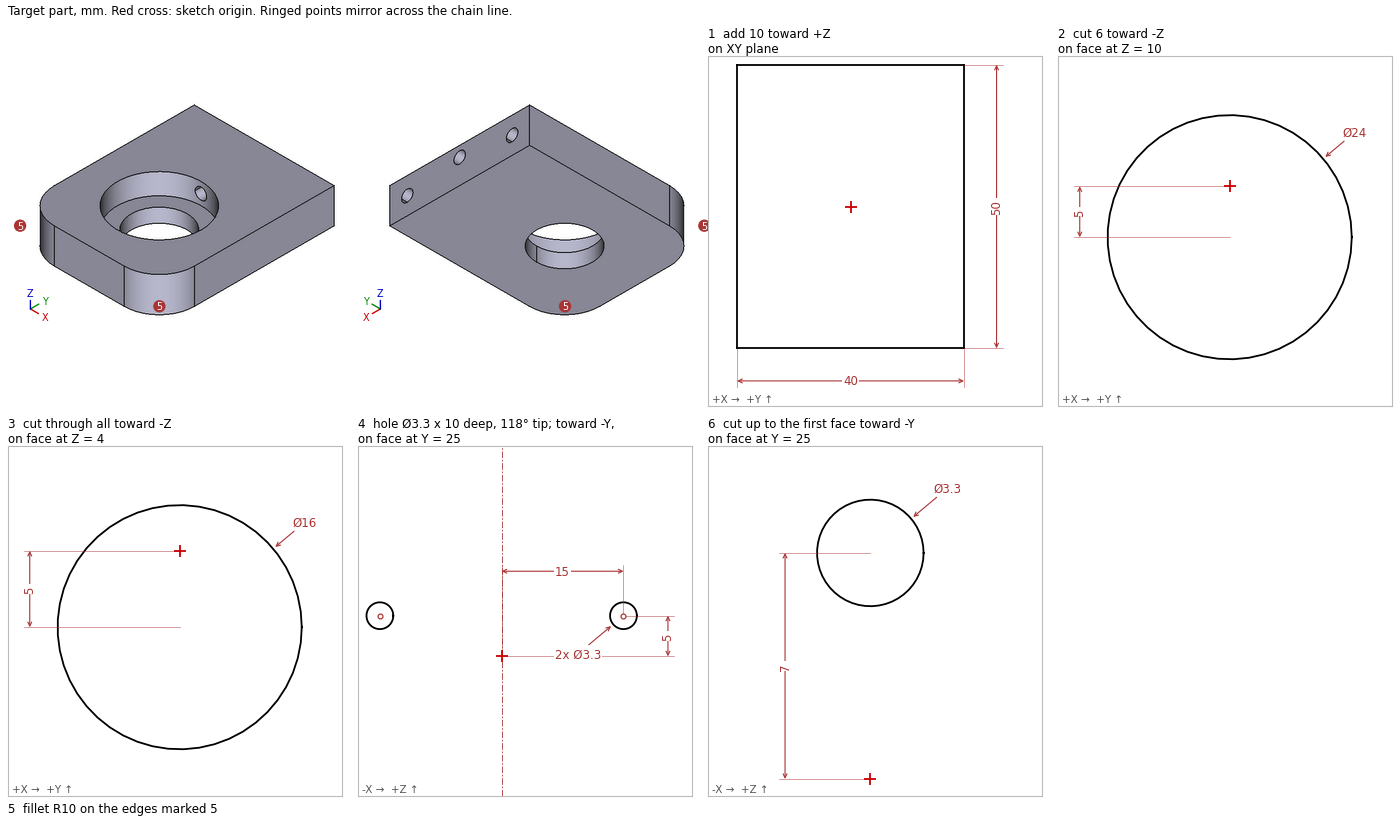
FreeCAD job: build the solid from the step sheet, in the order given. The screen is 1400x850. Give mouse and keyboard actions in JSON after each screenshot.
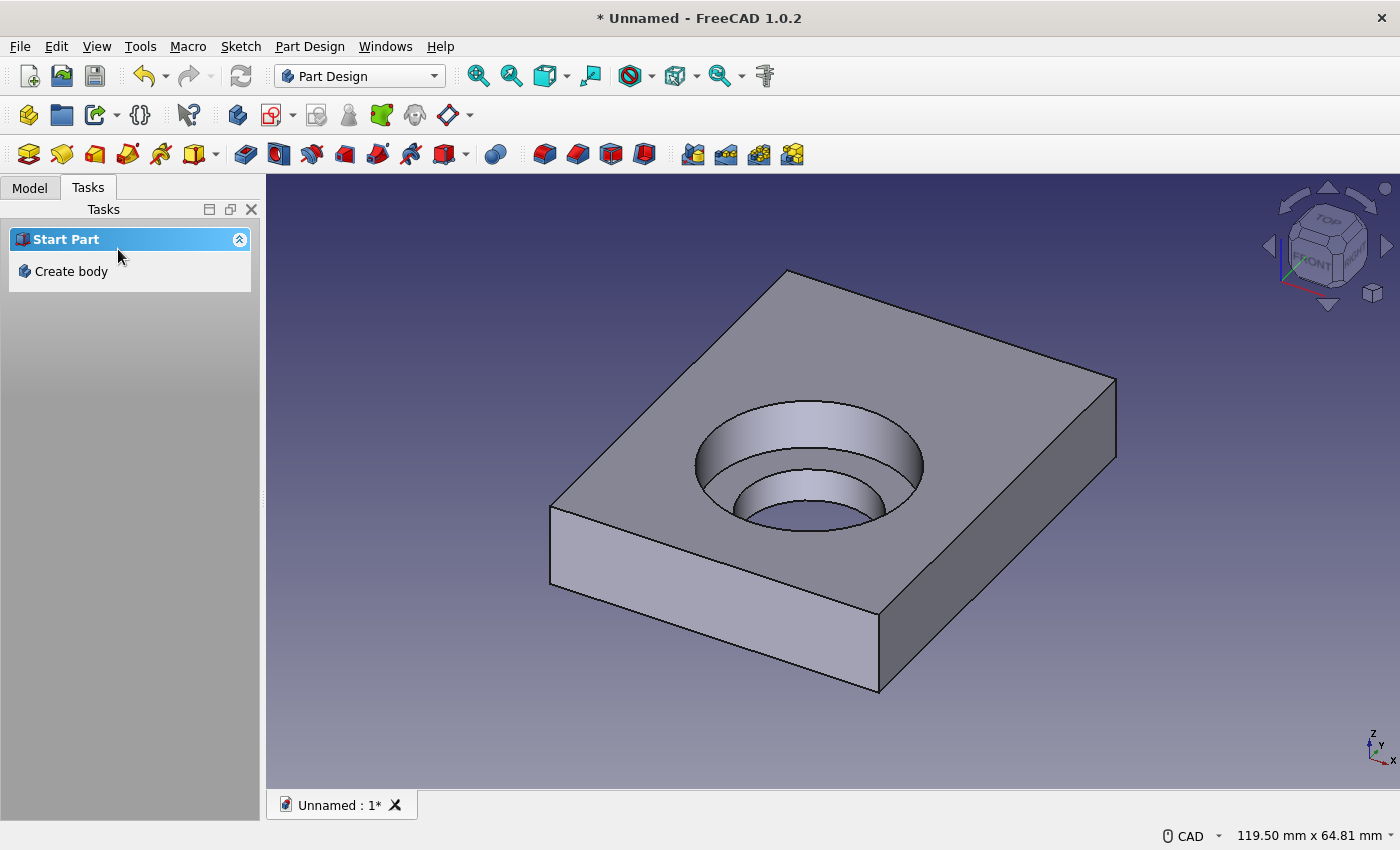
{"action": "key", "text": "4"}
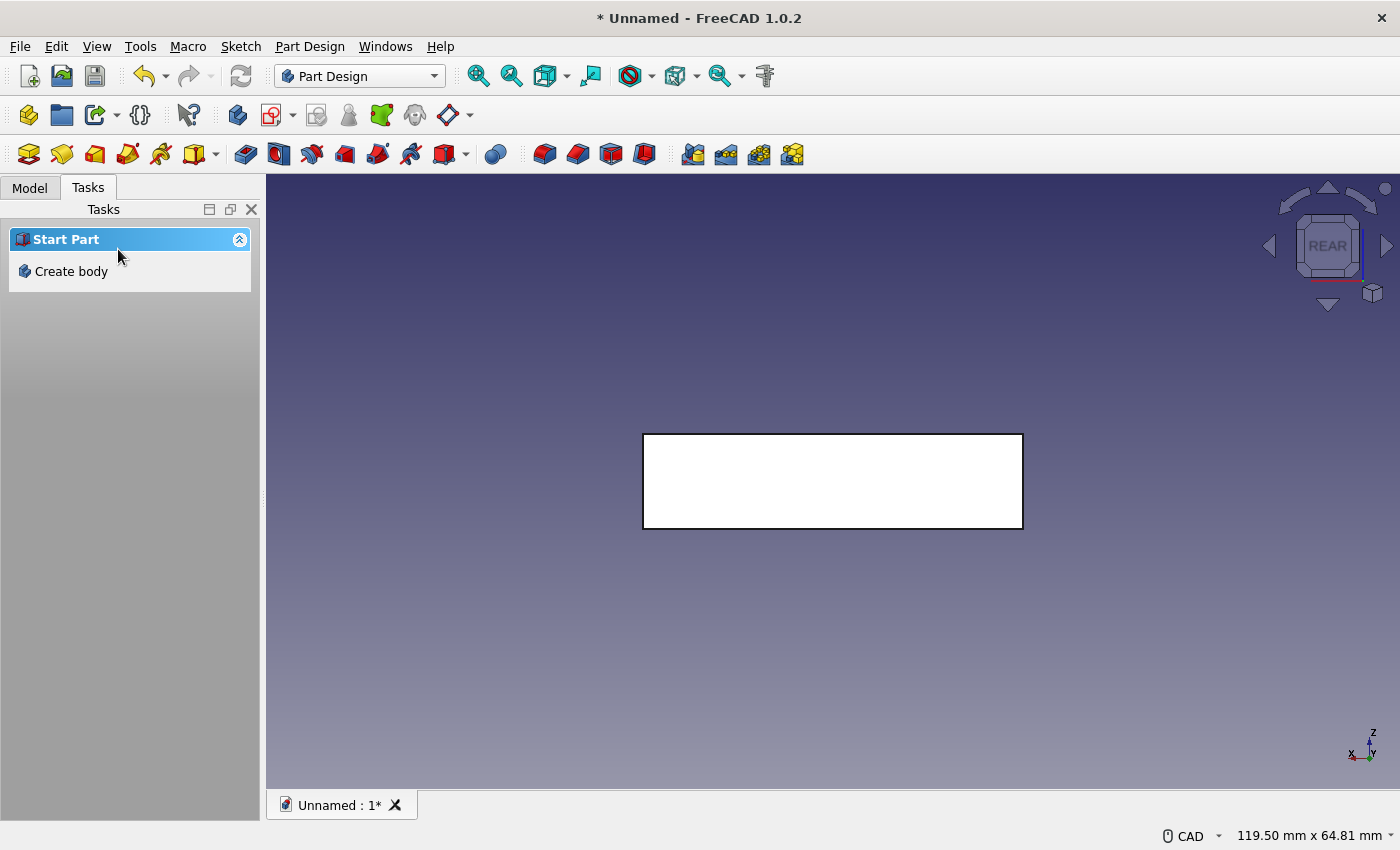
{"action": "left_click", "coordinate": [479, 76]}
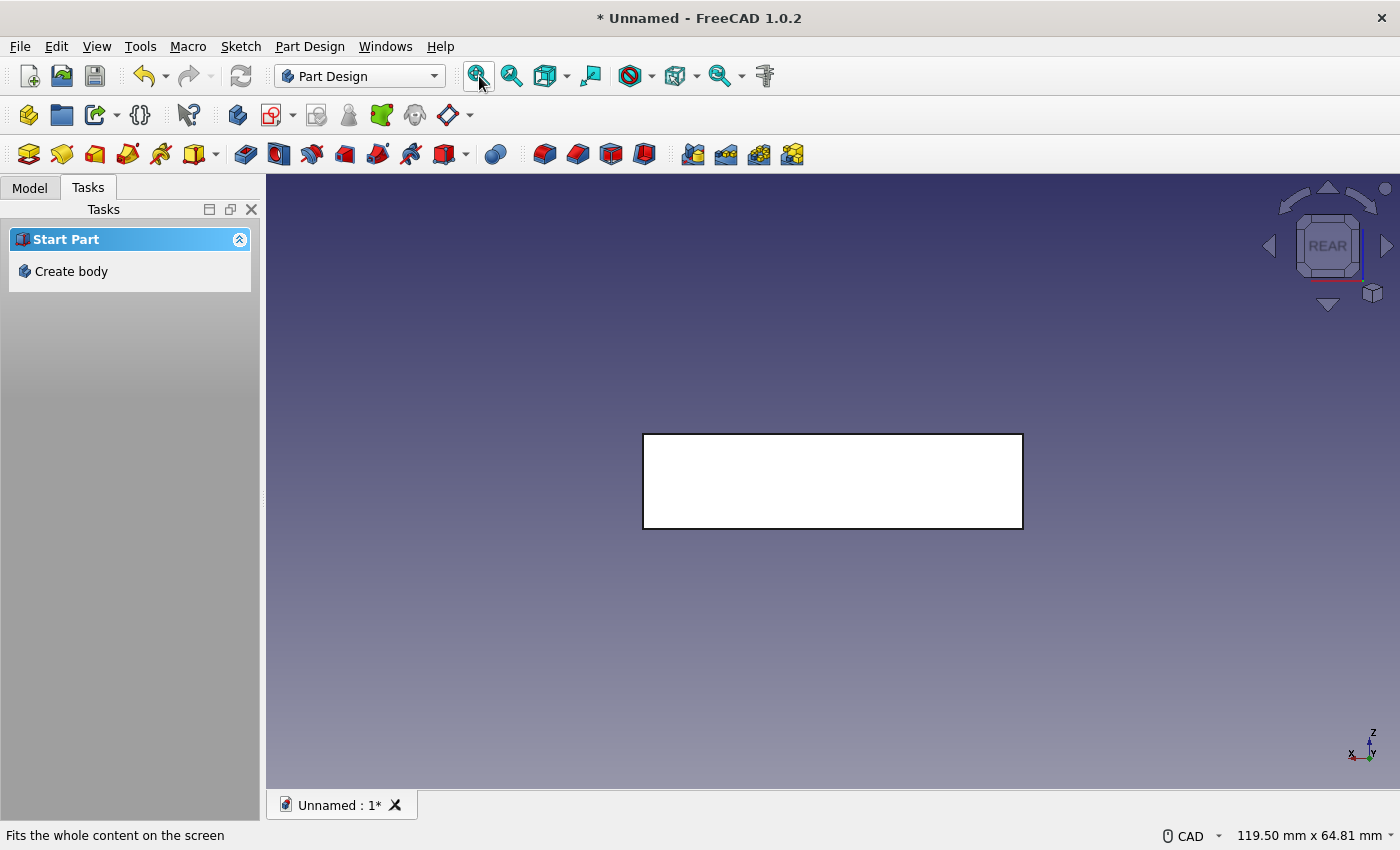
{"action": "left_click", "coordinate": [725, 481]}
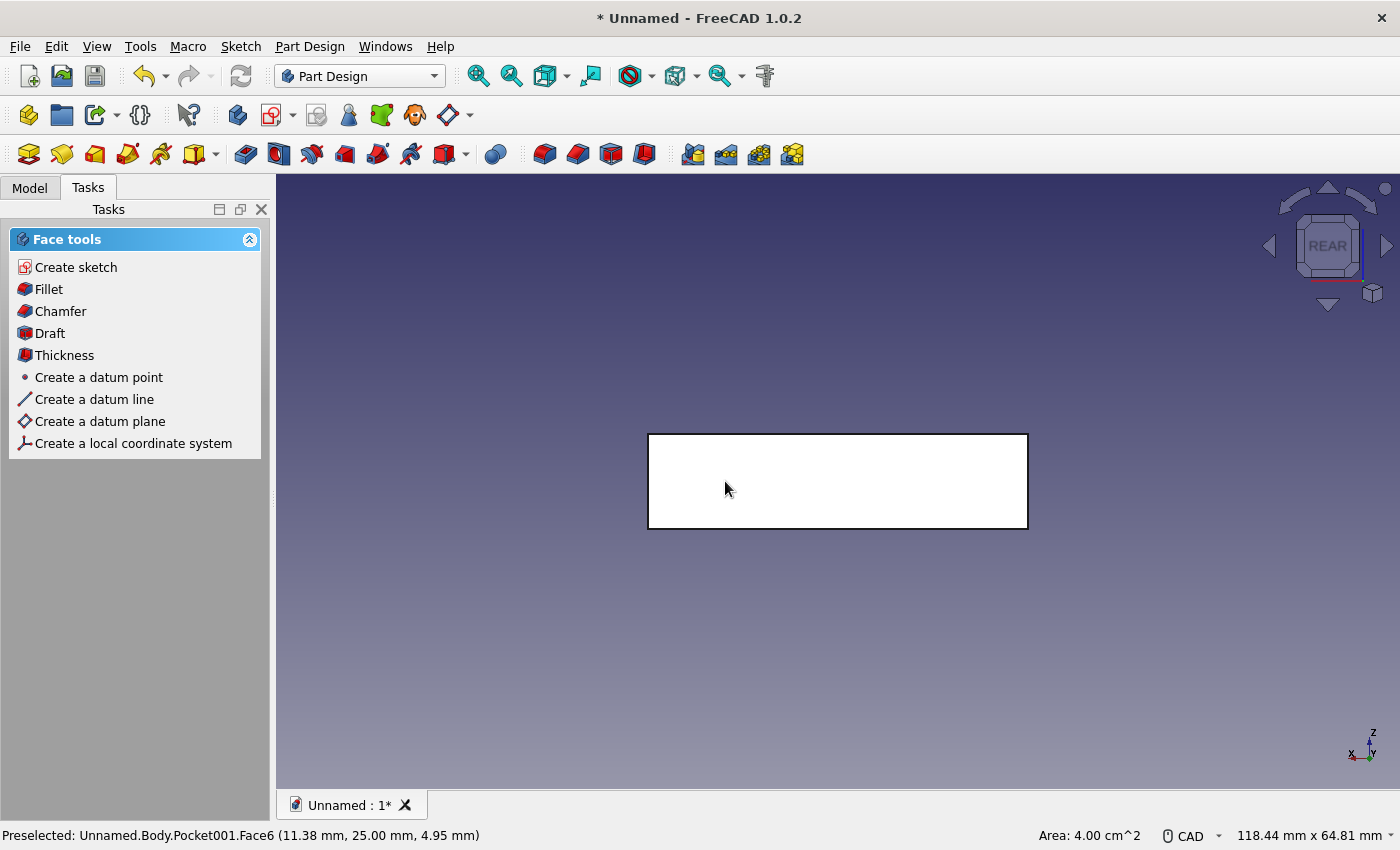
{"action": "left_click", "coordinate": [270, 116]}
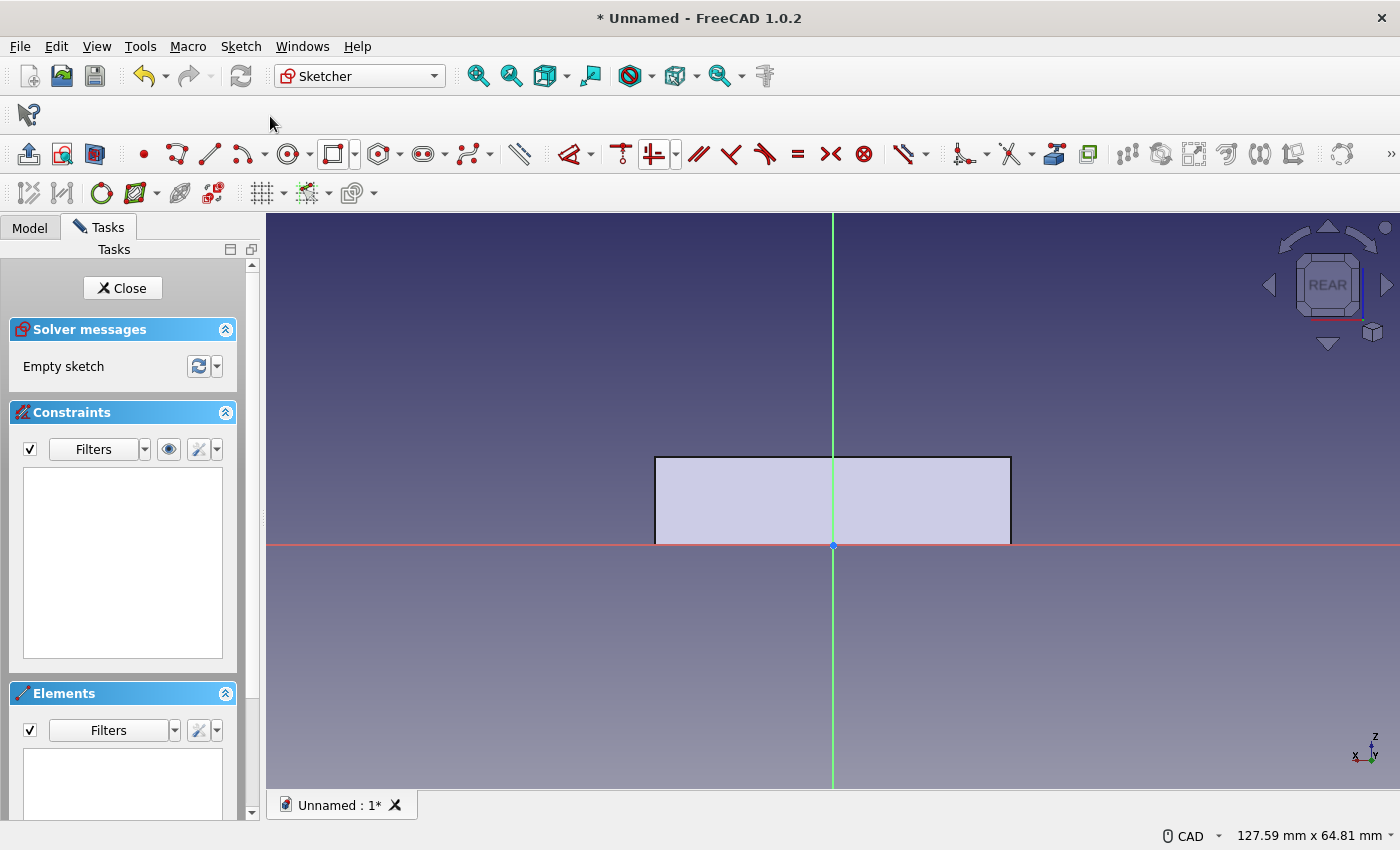
{"action": "scroll", "coordinate": [889, 528], "scroll_direction": "up", "scroll_amount": 4}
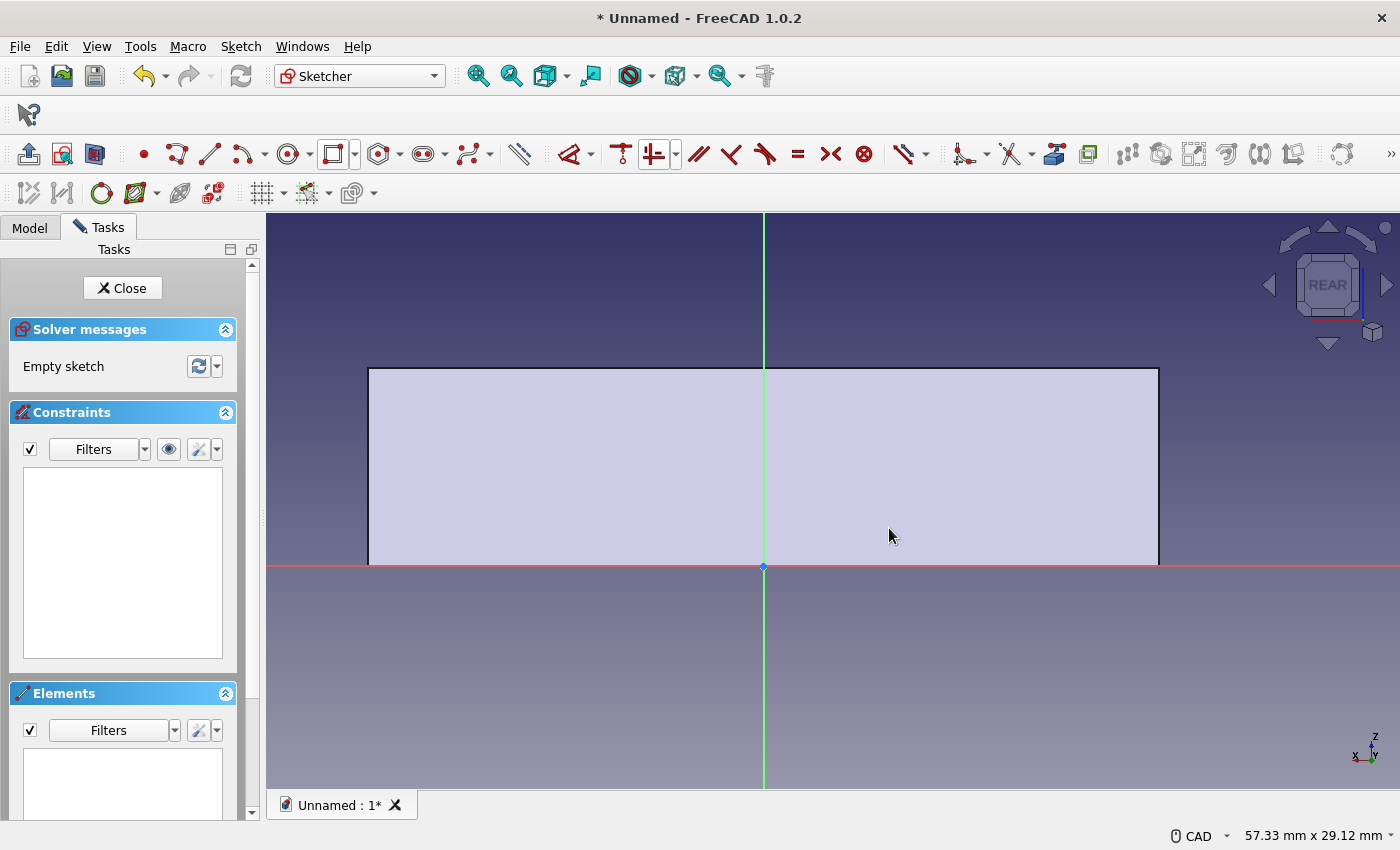
{"action": "left_click", "coordinate": [288, 154]}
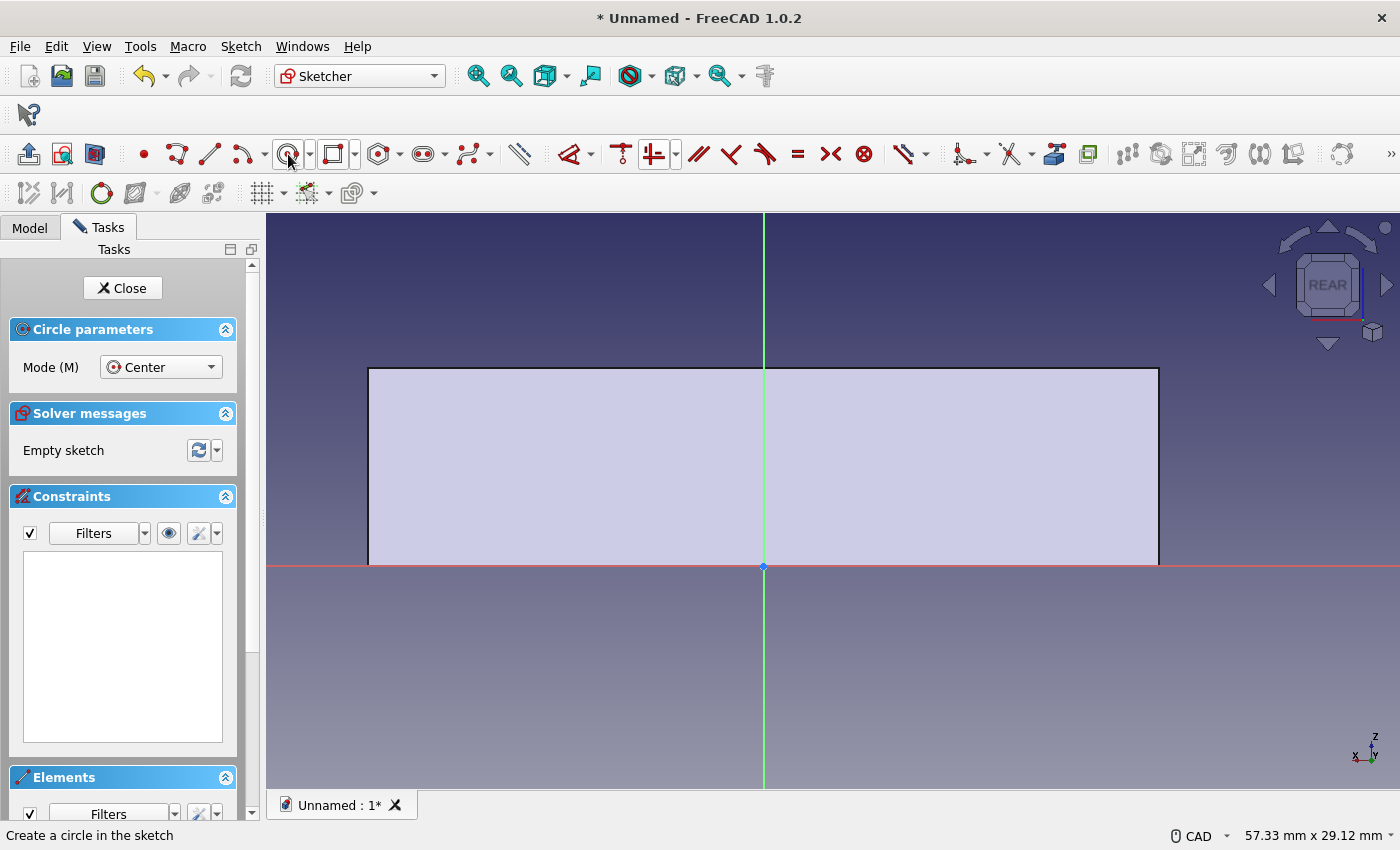
{"action": "left_click", "coordinate": [1060, 467]}
{"action": "mouse_move", "coordinate": [1083, 444]}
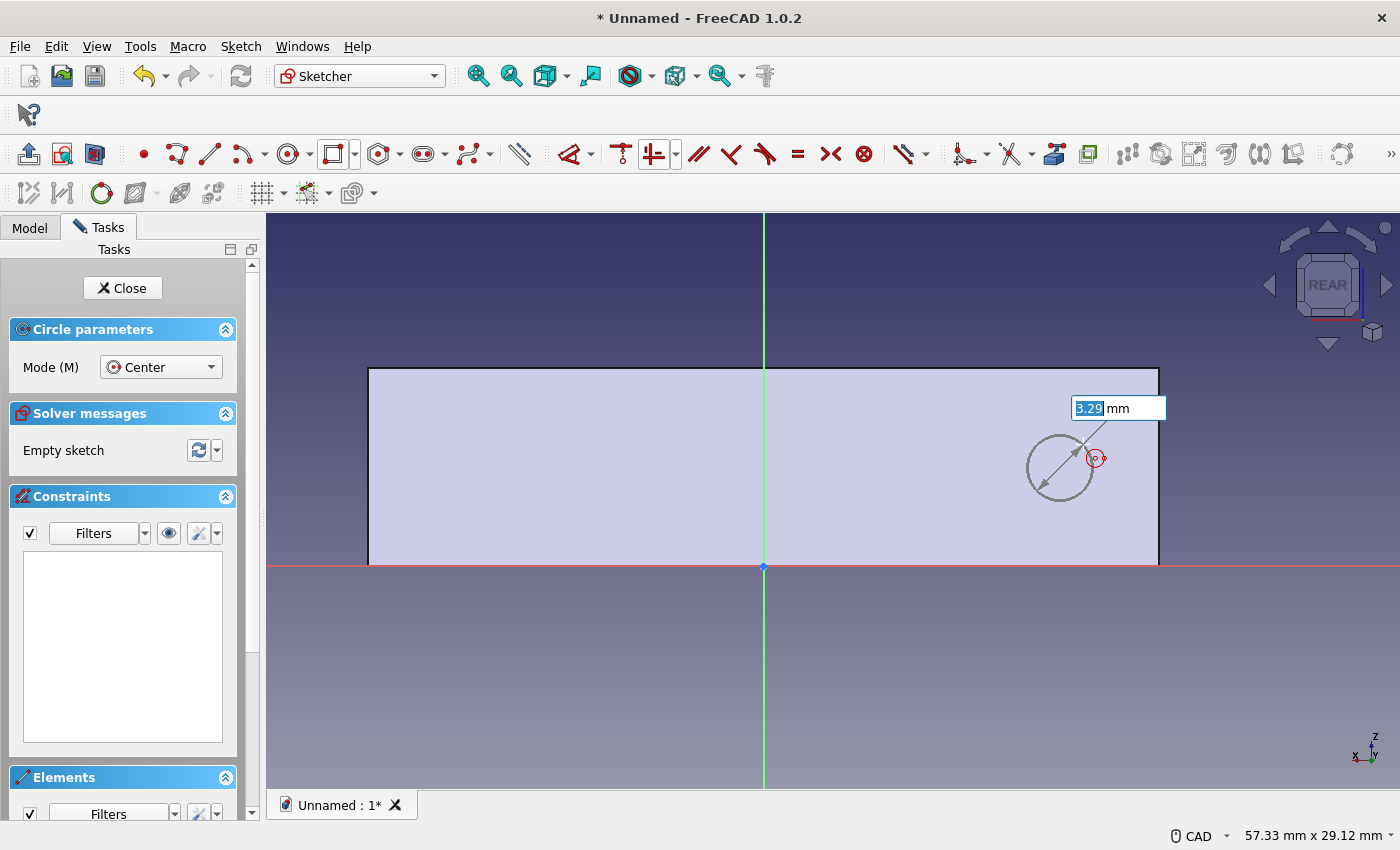
{"action": "type", "text": "3.3"}
{"action": "key", "text": "Return"}